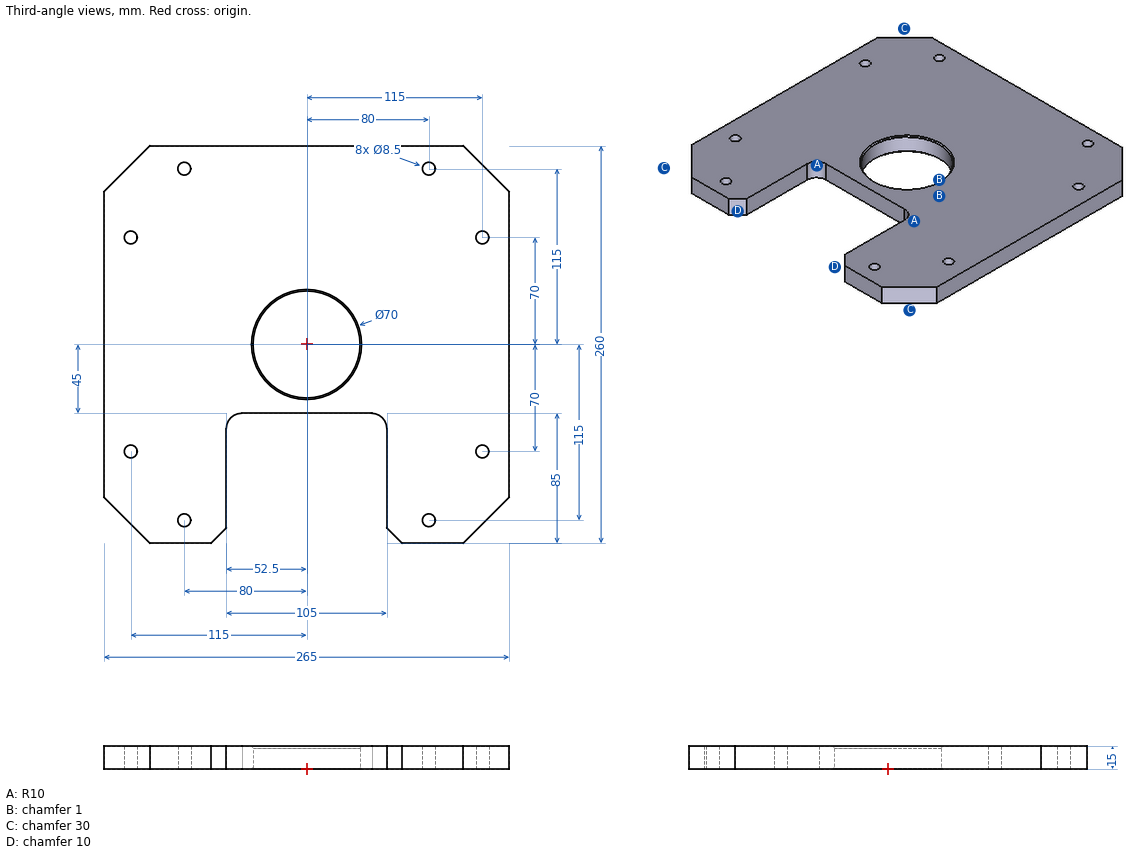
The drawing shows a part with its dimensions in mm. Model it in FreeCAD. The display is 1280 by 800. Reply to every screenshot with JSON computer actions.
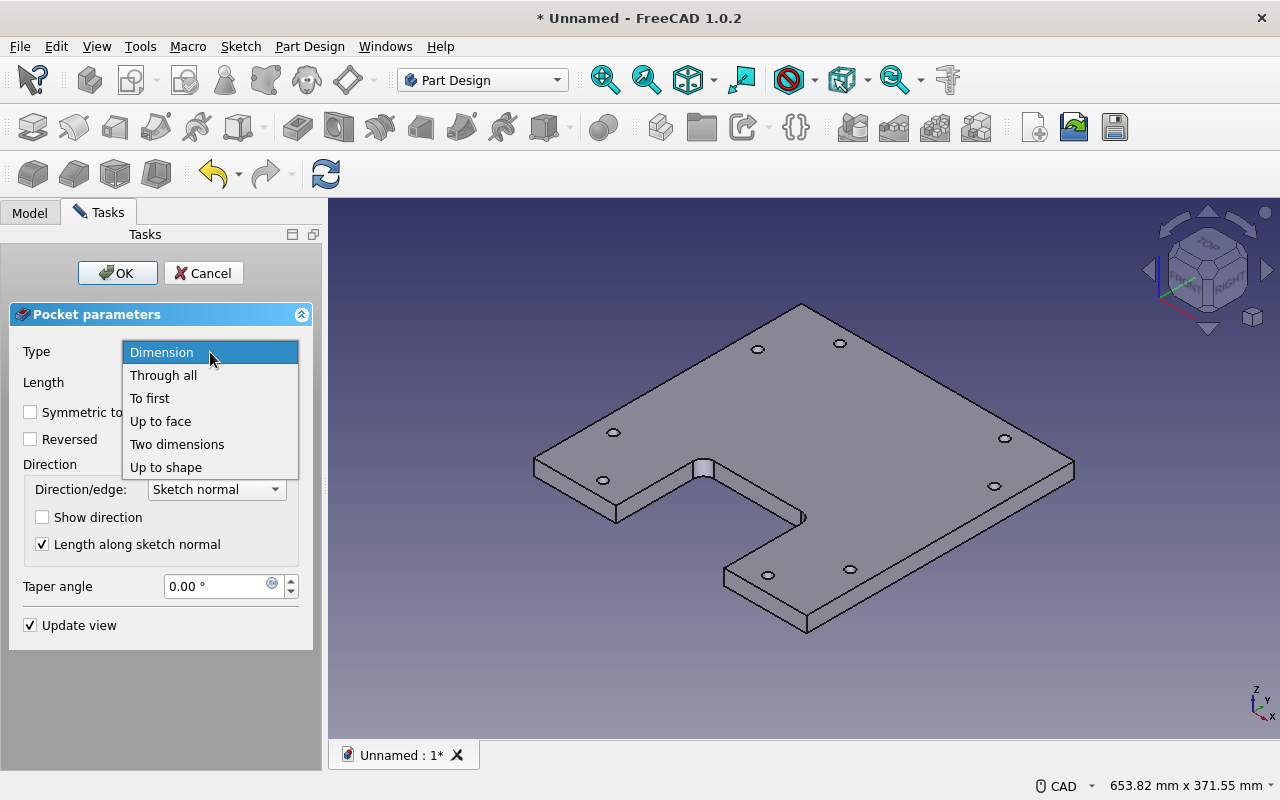
{"action": "left_click", "coordinate": [208, 376]}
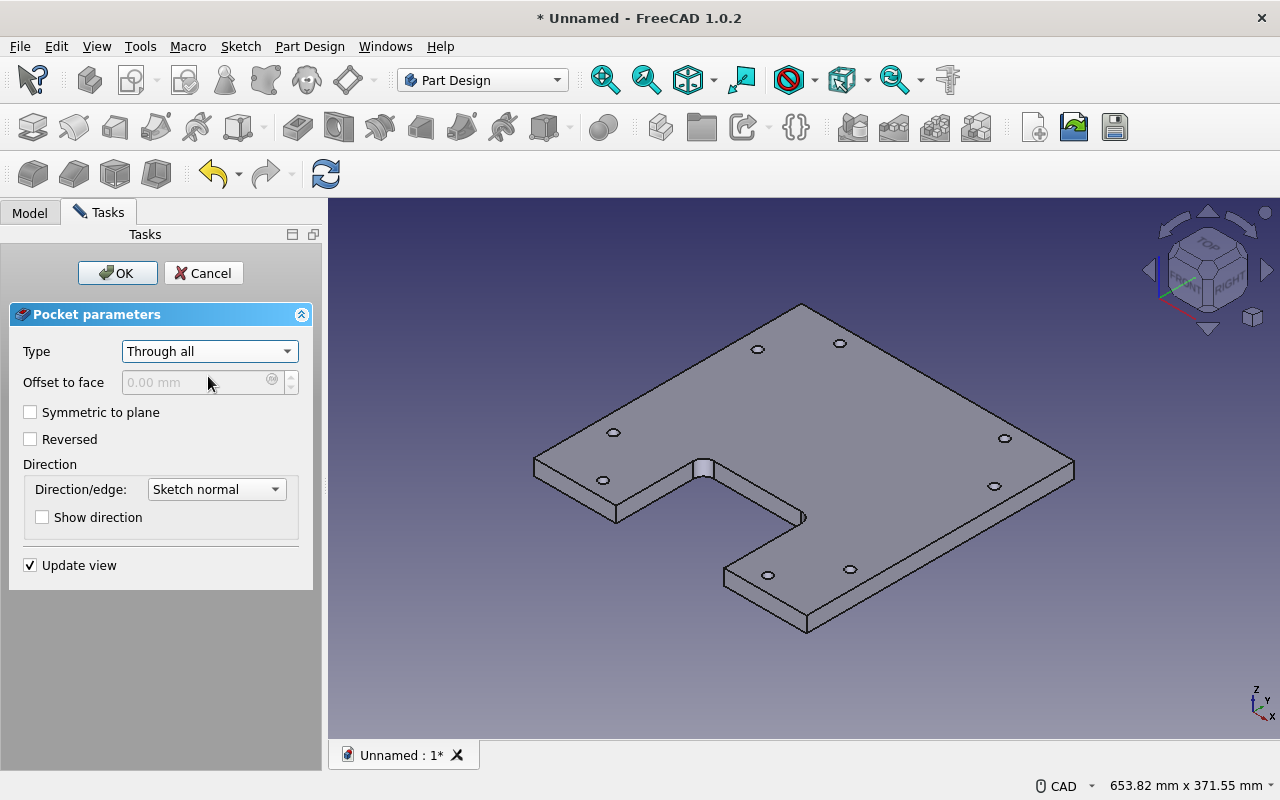
{"action": "left_click", "coordinate": [31, 439]}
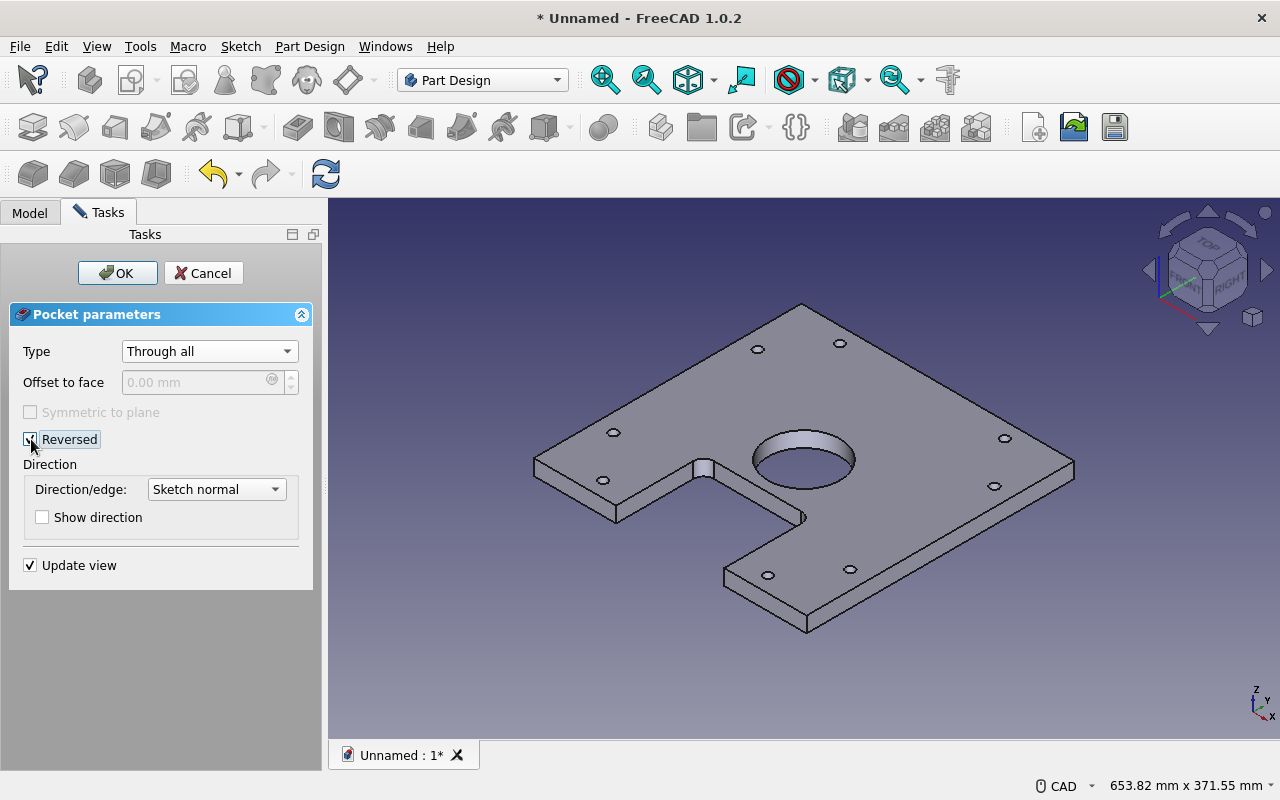
{"action": "left_click", "coordinate": [118, 273]}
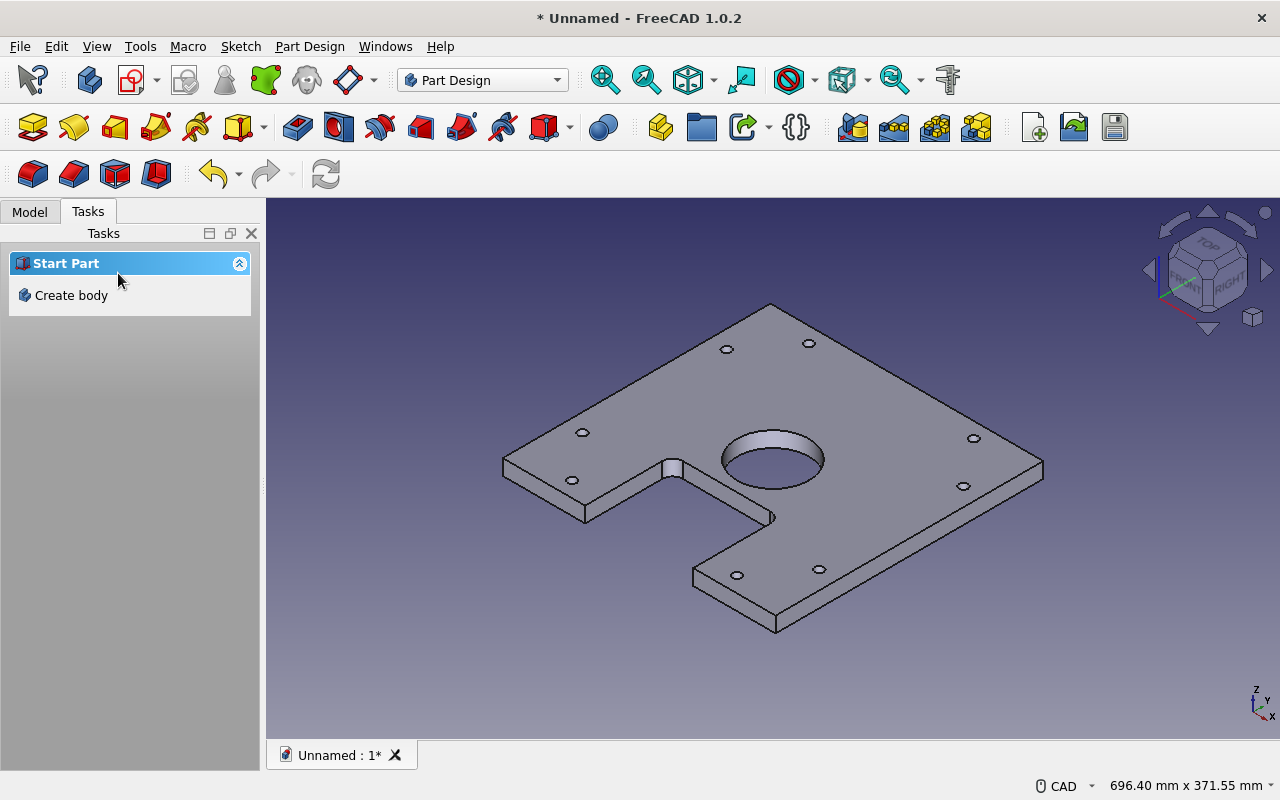
{"action": "left_click", "coordinate": [737, 438]}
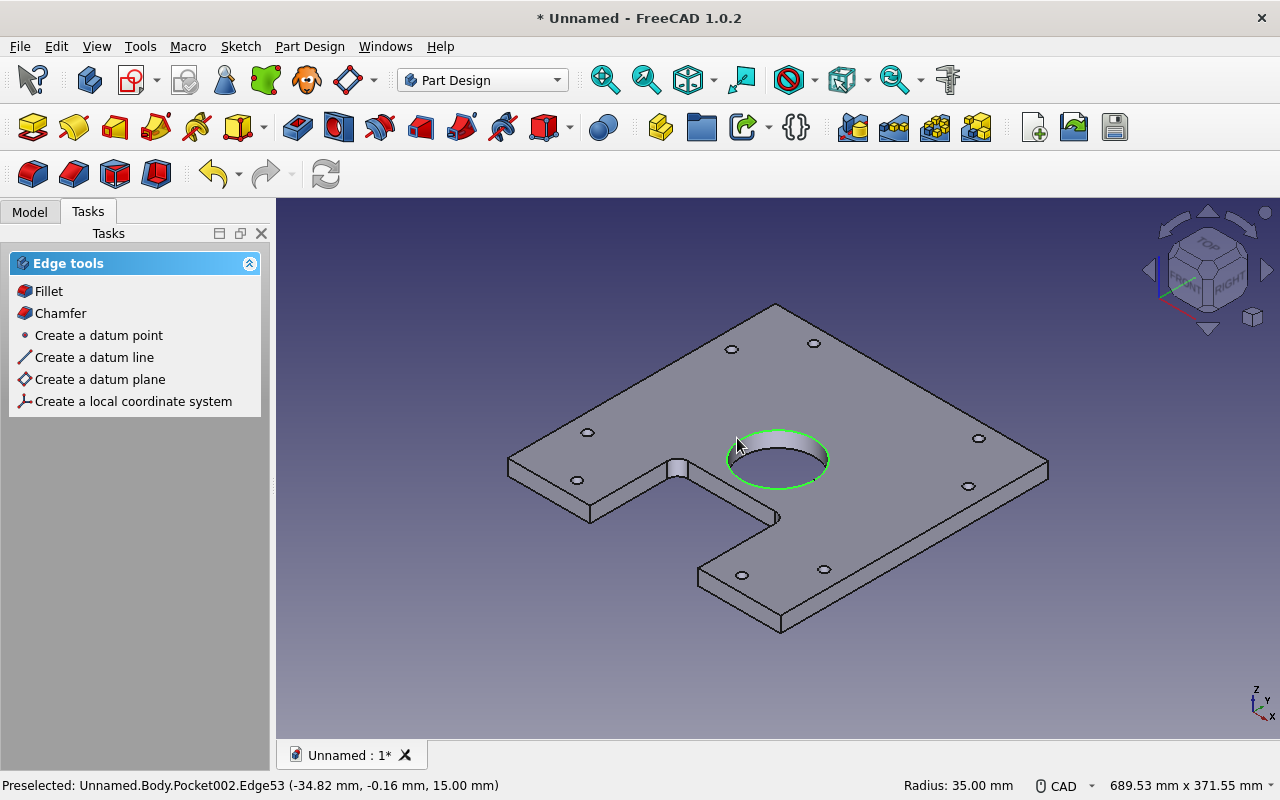
{"action": "key", "text": "2"}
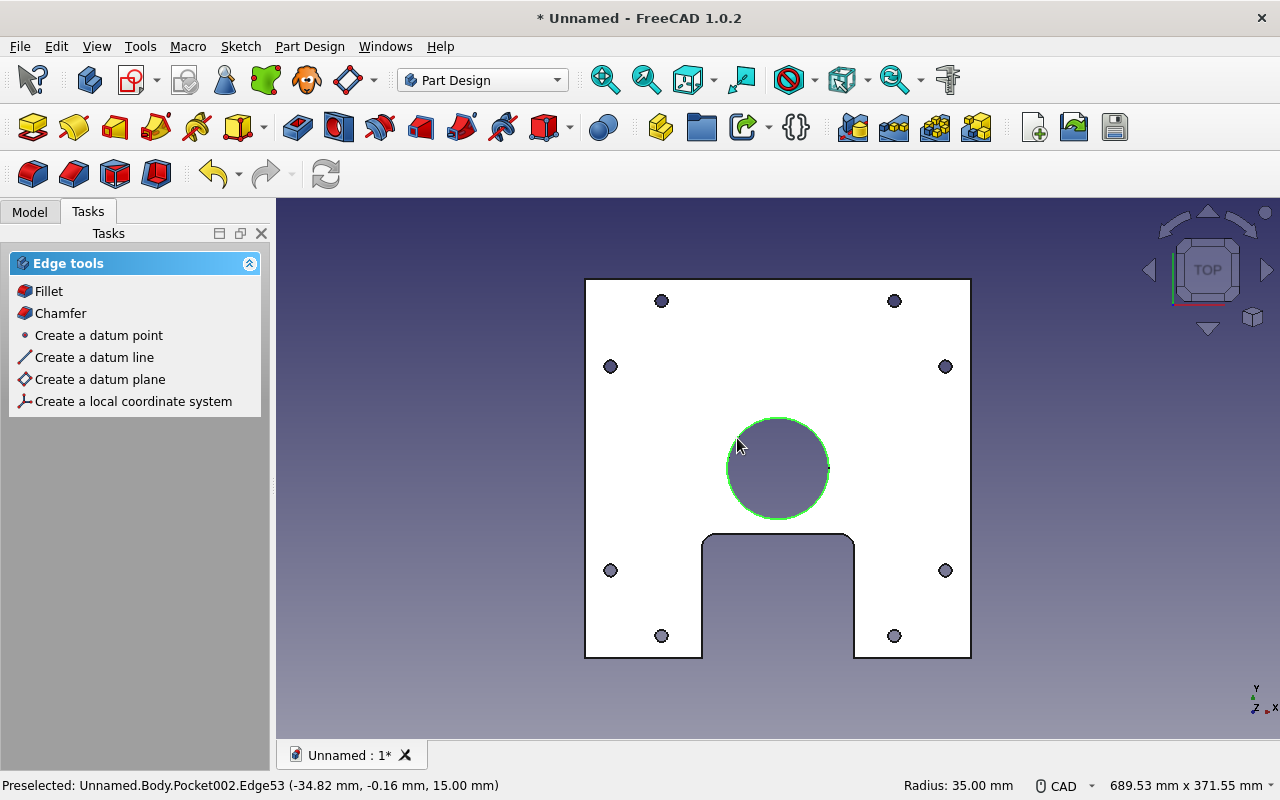
{"action": "key", "text": "0"}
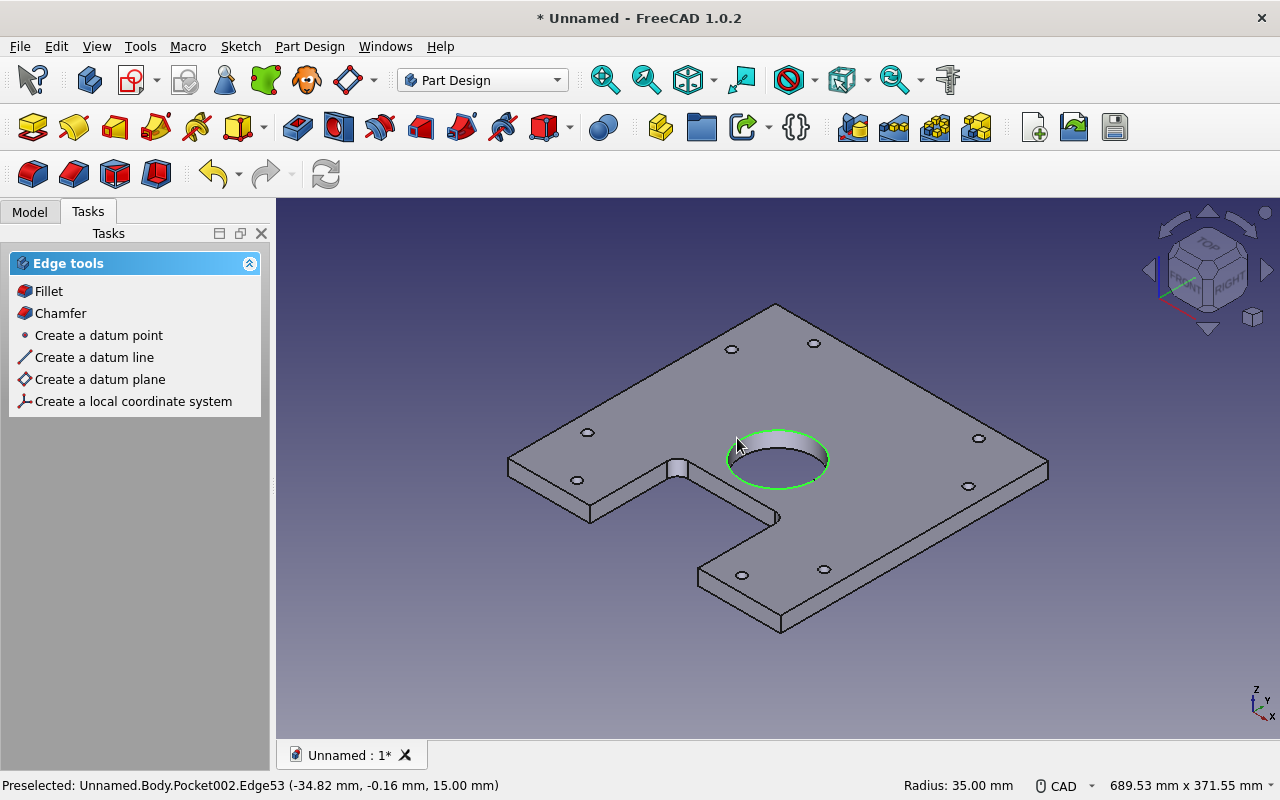
{"action": "key", "text": "1"}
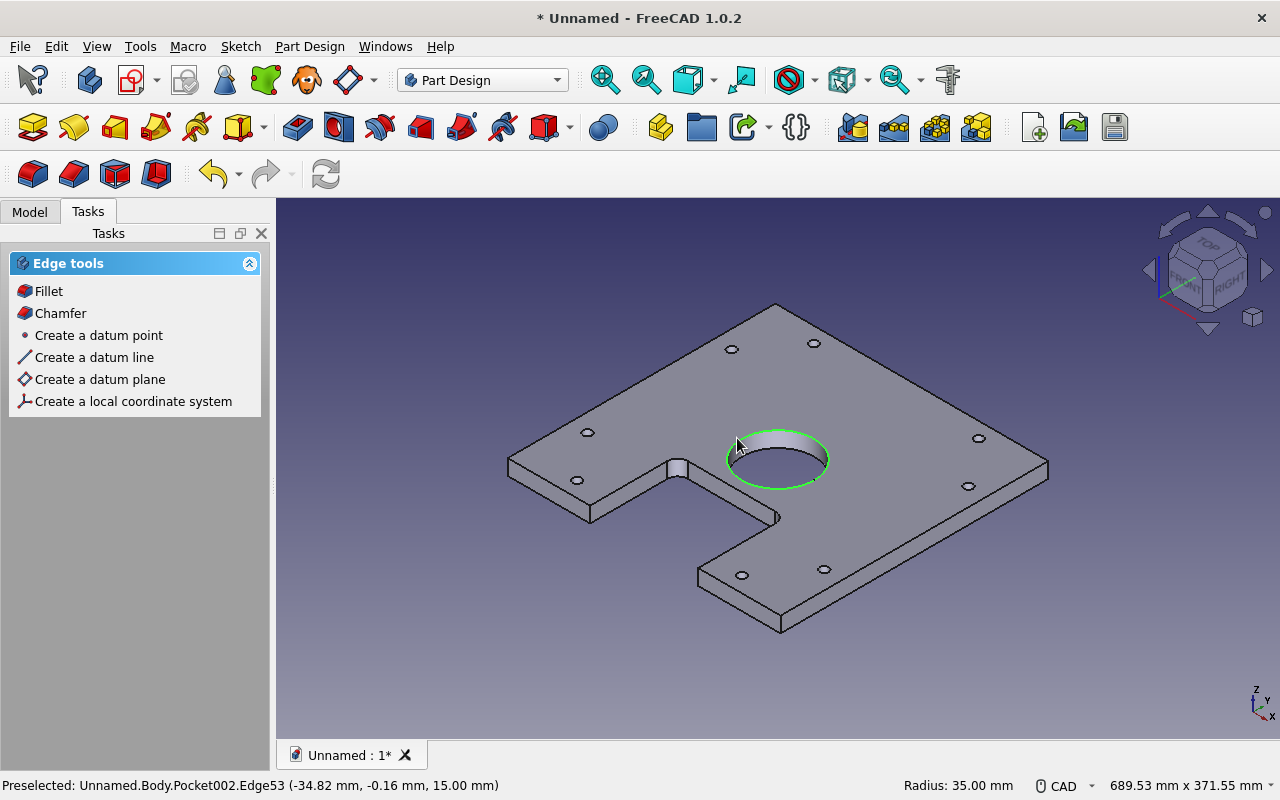
{"action": "left_click", "coordinate": [606, 80]}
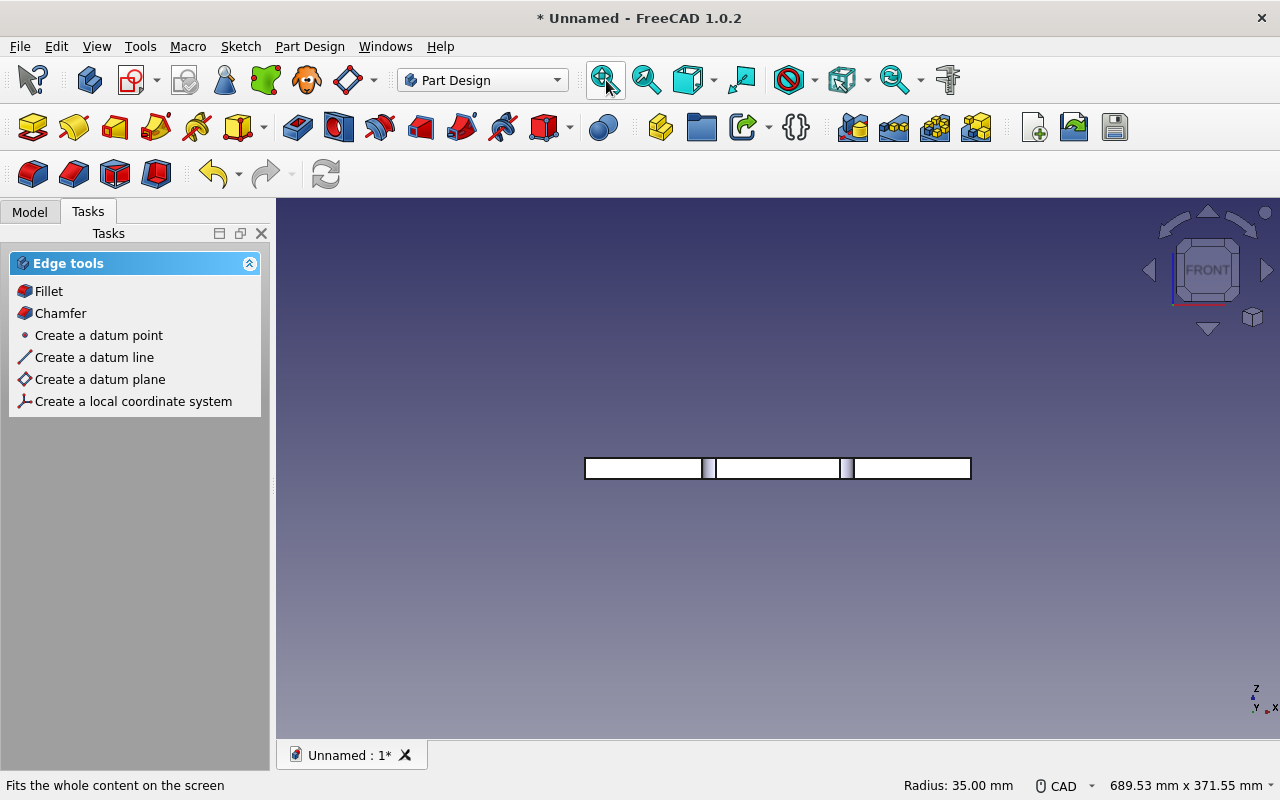
{"action": "key", "text": "3"}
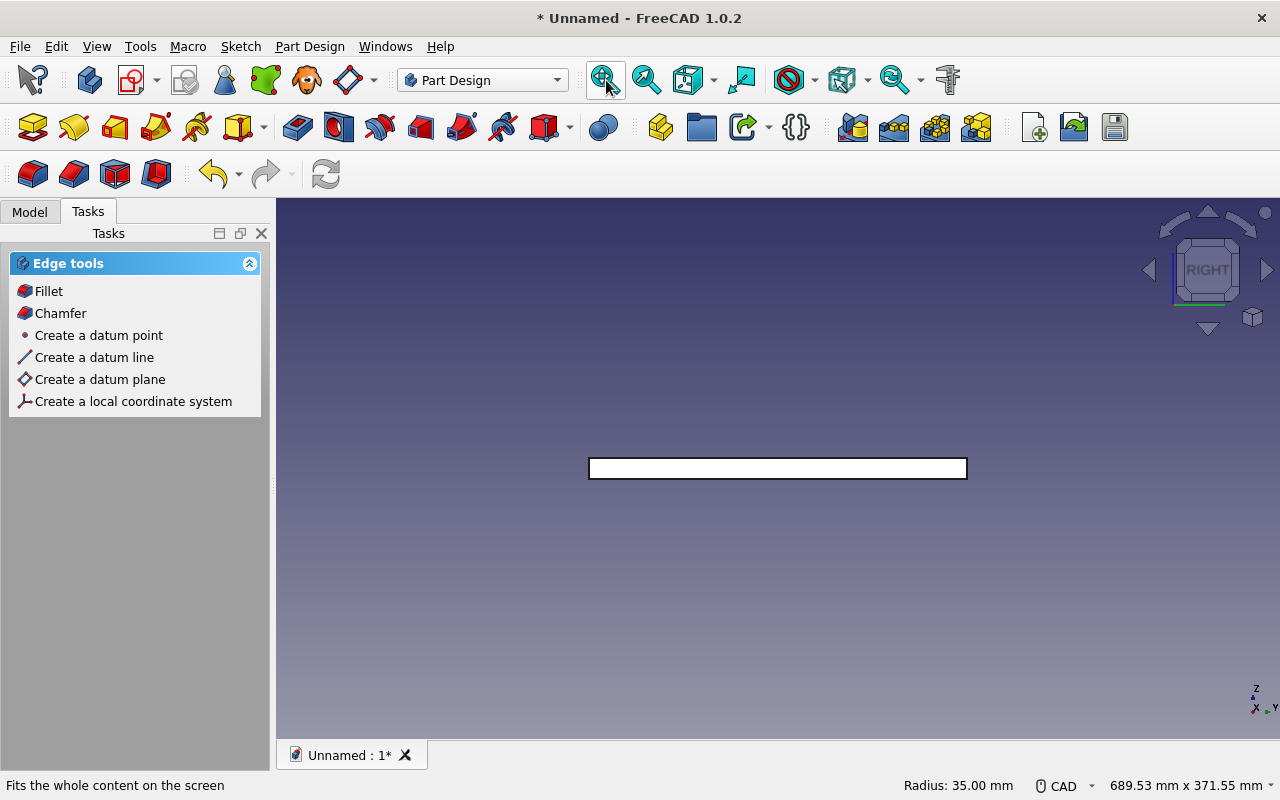
{"action": "key", "text": "v f"}